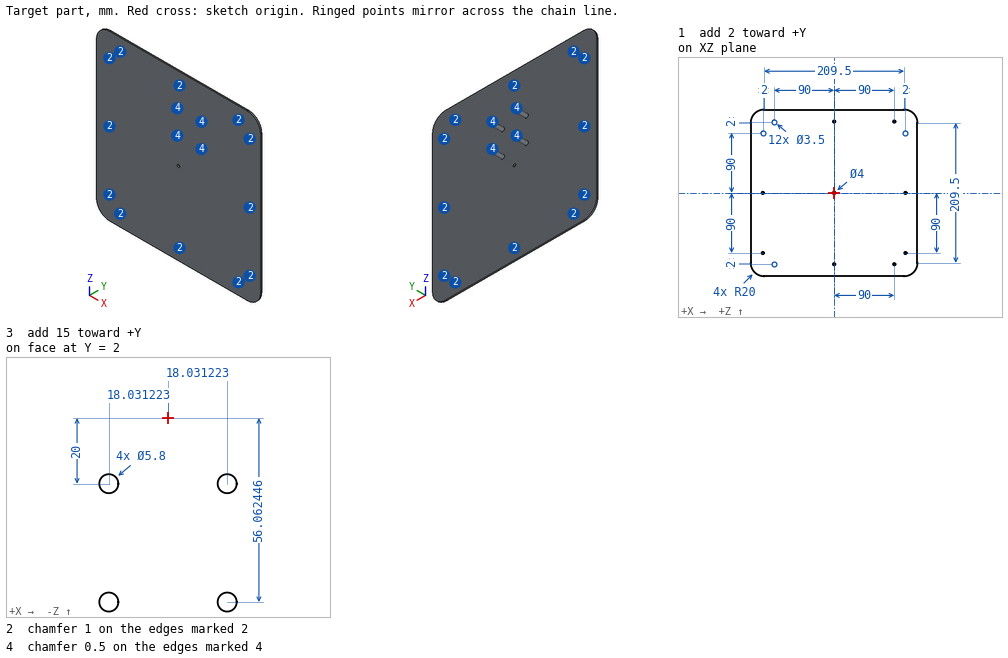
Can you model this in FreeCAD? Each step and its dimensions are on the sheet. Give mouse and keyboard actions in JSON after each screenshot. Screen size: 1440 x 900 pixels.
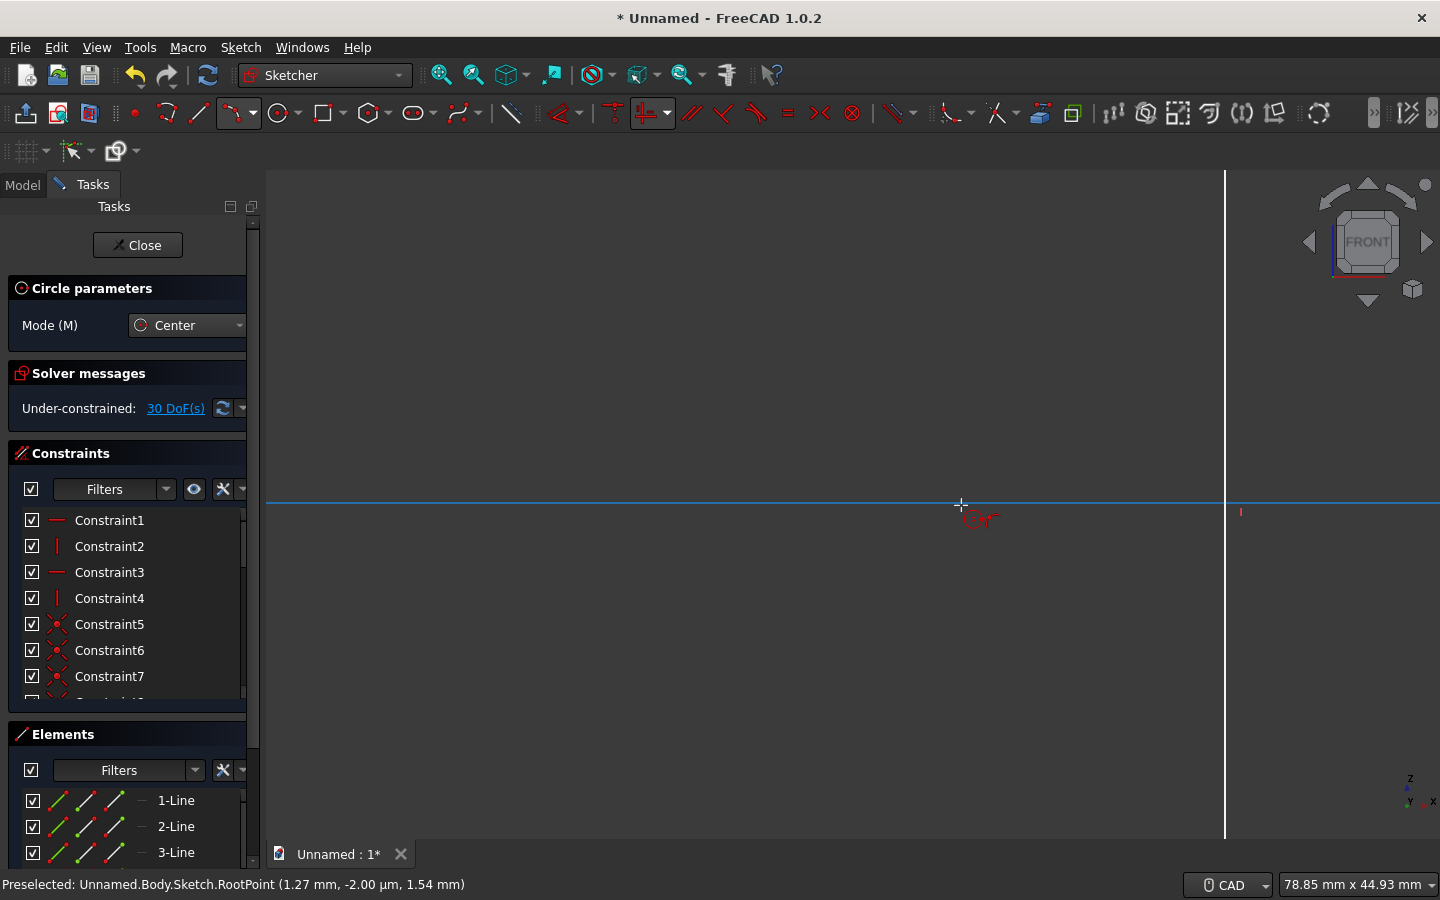
{"action": "scroll", "coordinate": [962, 505], "scroll_direction": "down", "scroll_amount": 11}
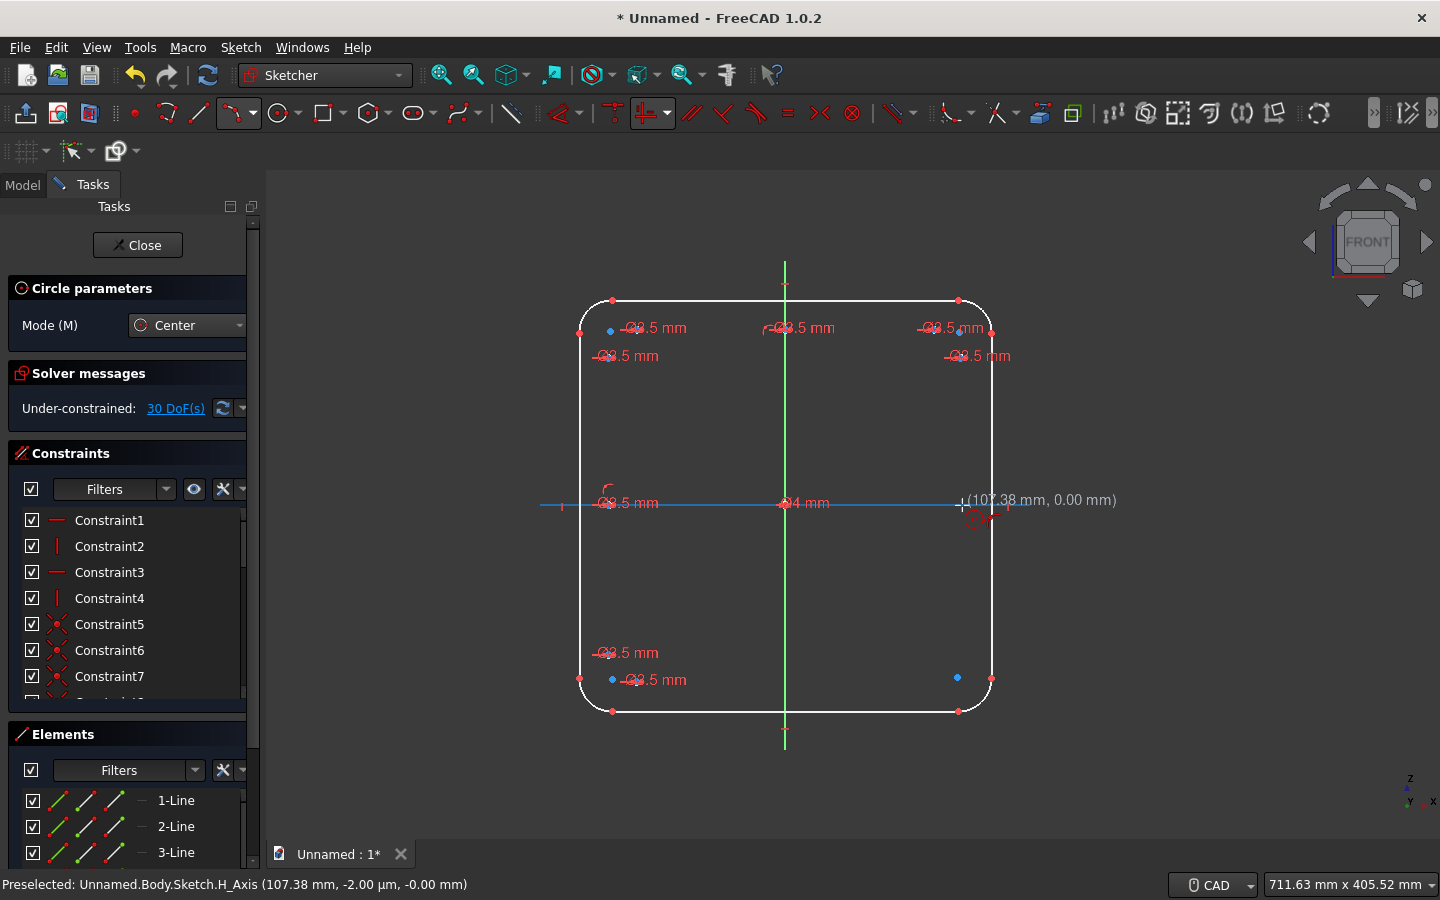
{"action": "left_click", "coordinate": [961, 505]}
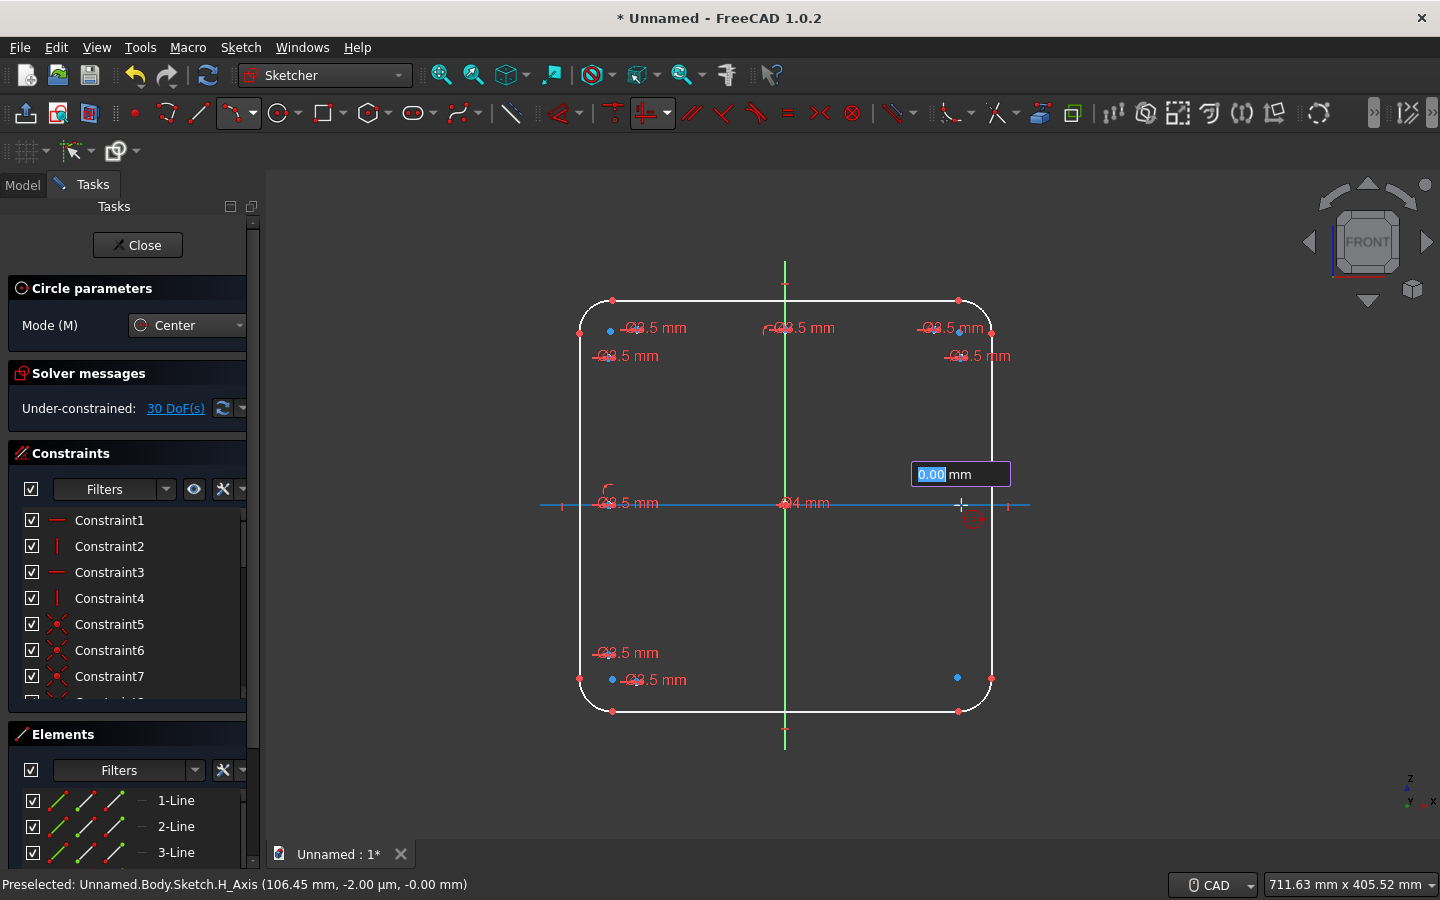
{"action": "scroll", "coordinate": [962, 502], "scroll_direction": "up", "scroll_amount": 9}
{"action": "mouse_move", "coordinate": [962, 502]}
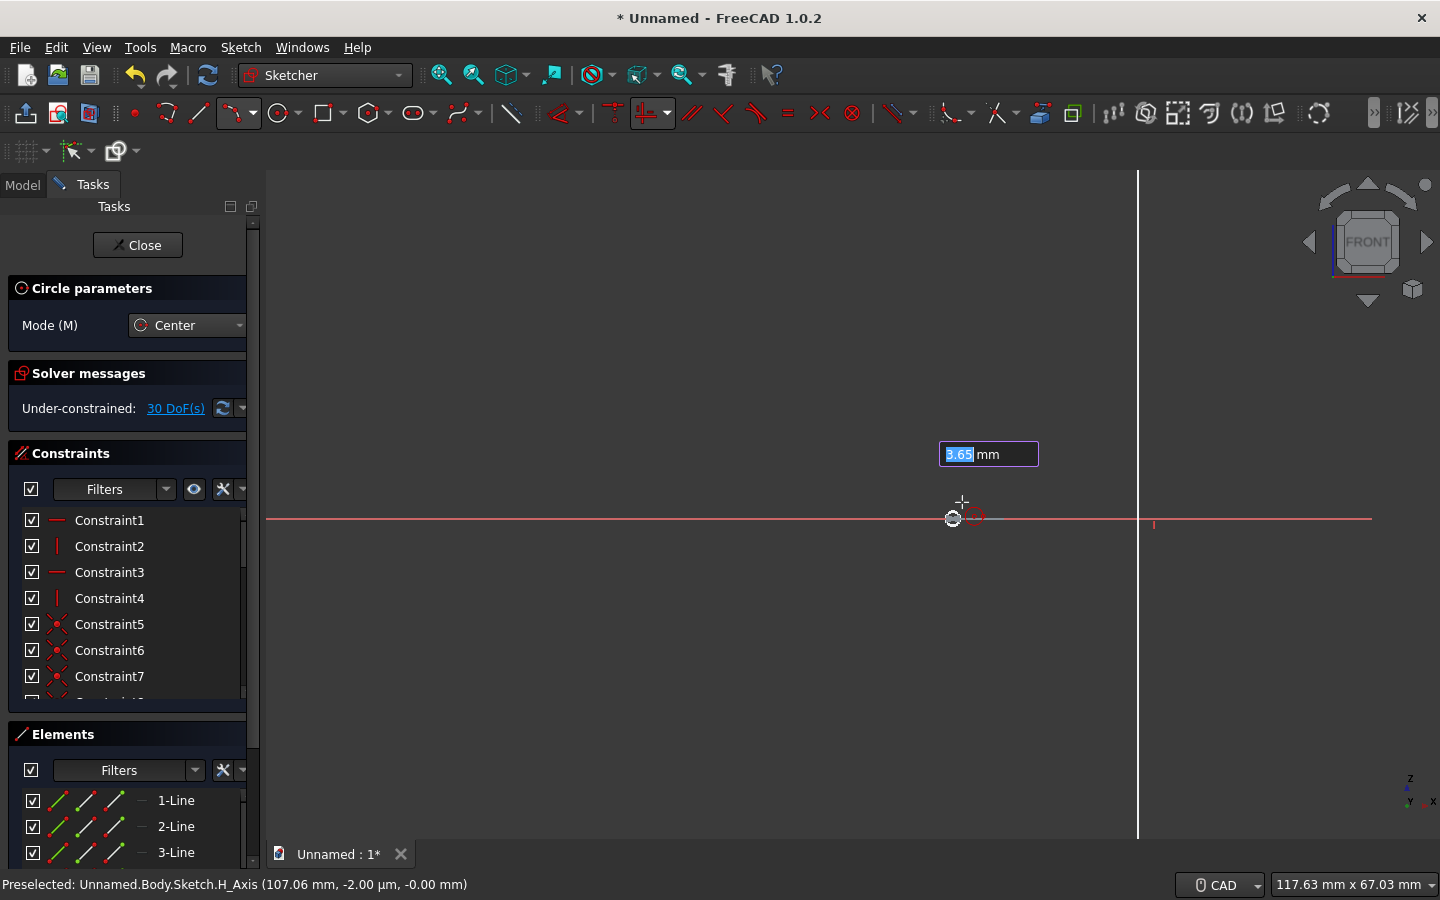
{"action": "type", "text": "3.5"}
{"action": "key", "text": "Return"}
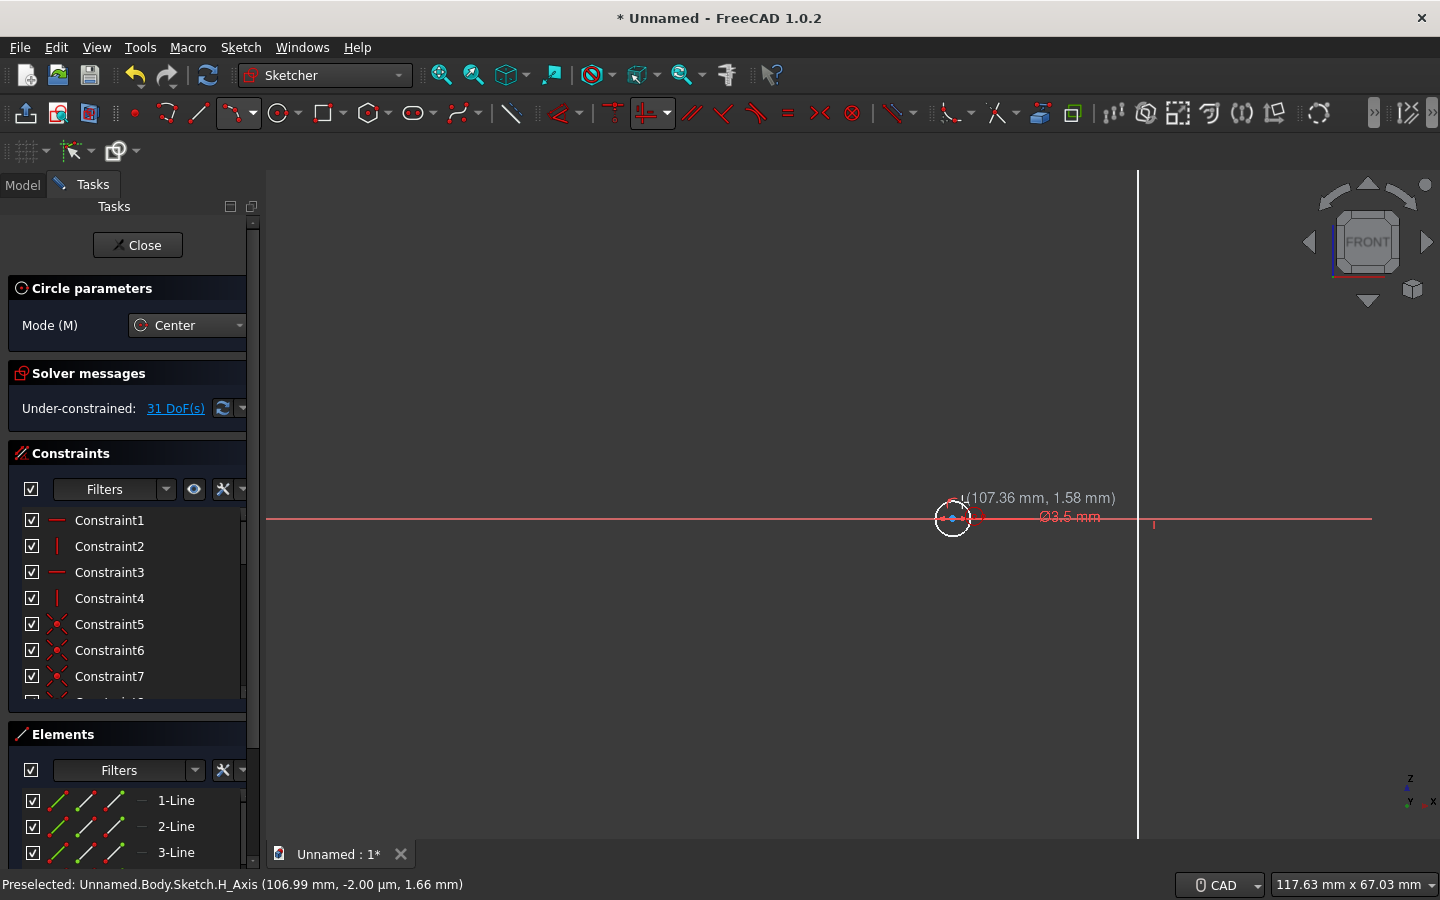
{"action": "scroll", "coordinate": [962, 502], "scroll_direction": "down", "scroll_amount": 9}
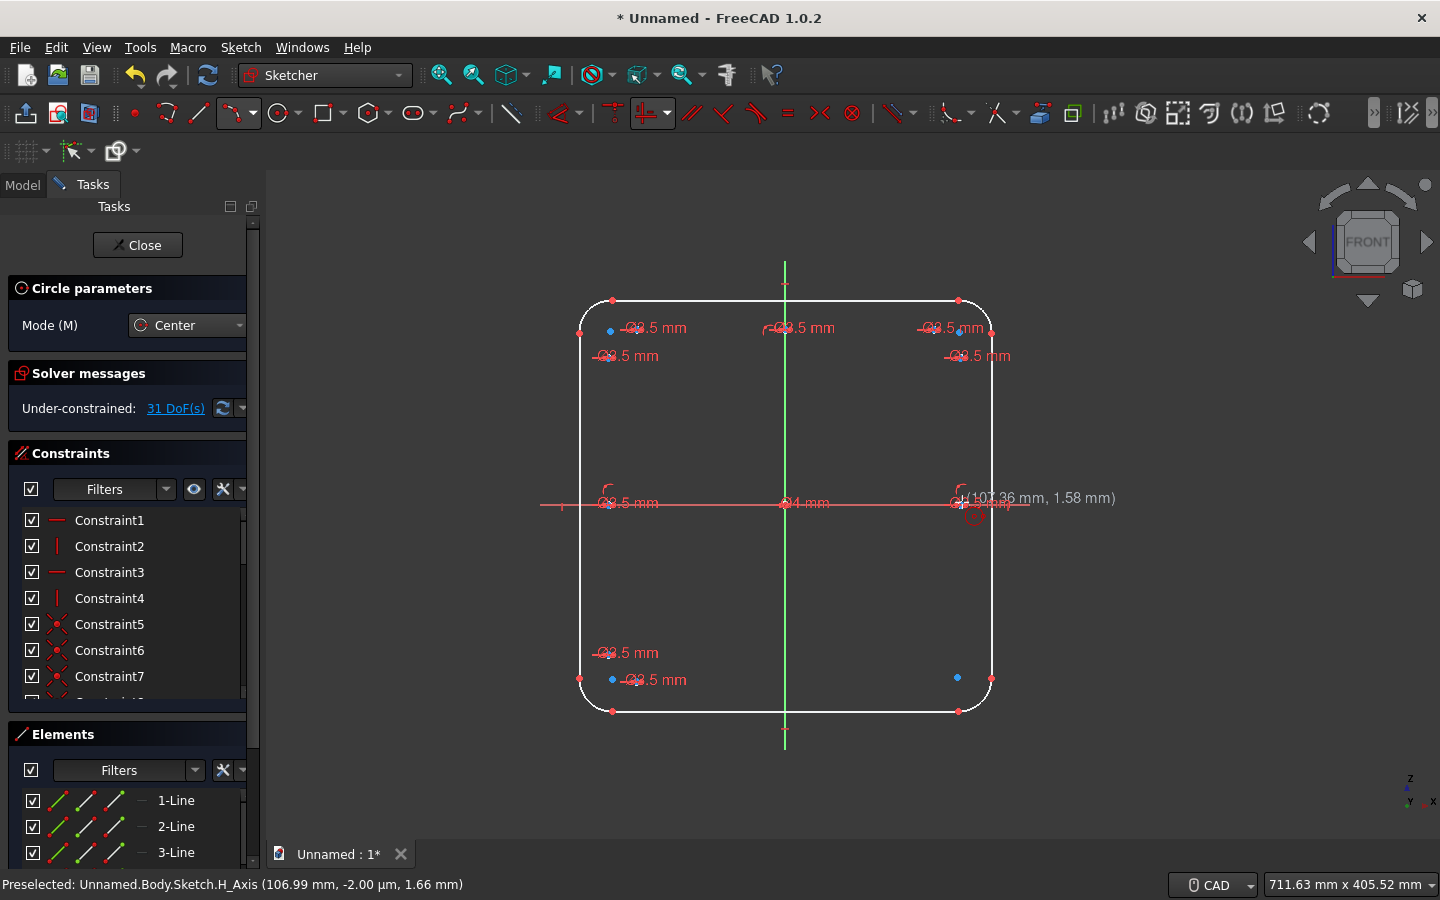
{"action": "scroll", "coordinate": [785, 681], "scroll_direction": "up", "scroll_amount": 11}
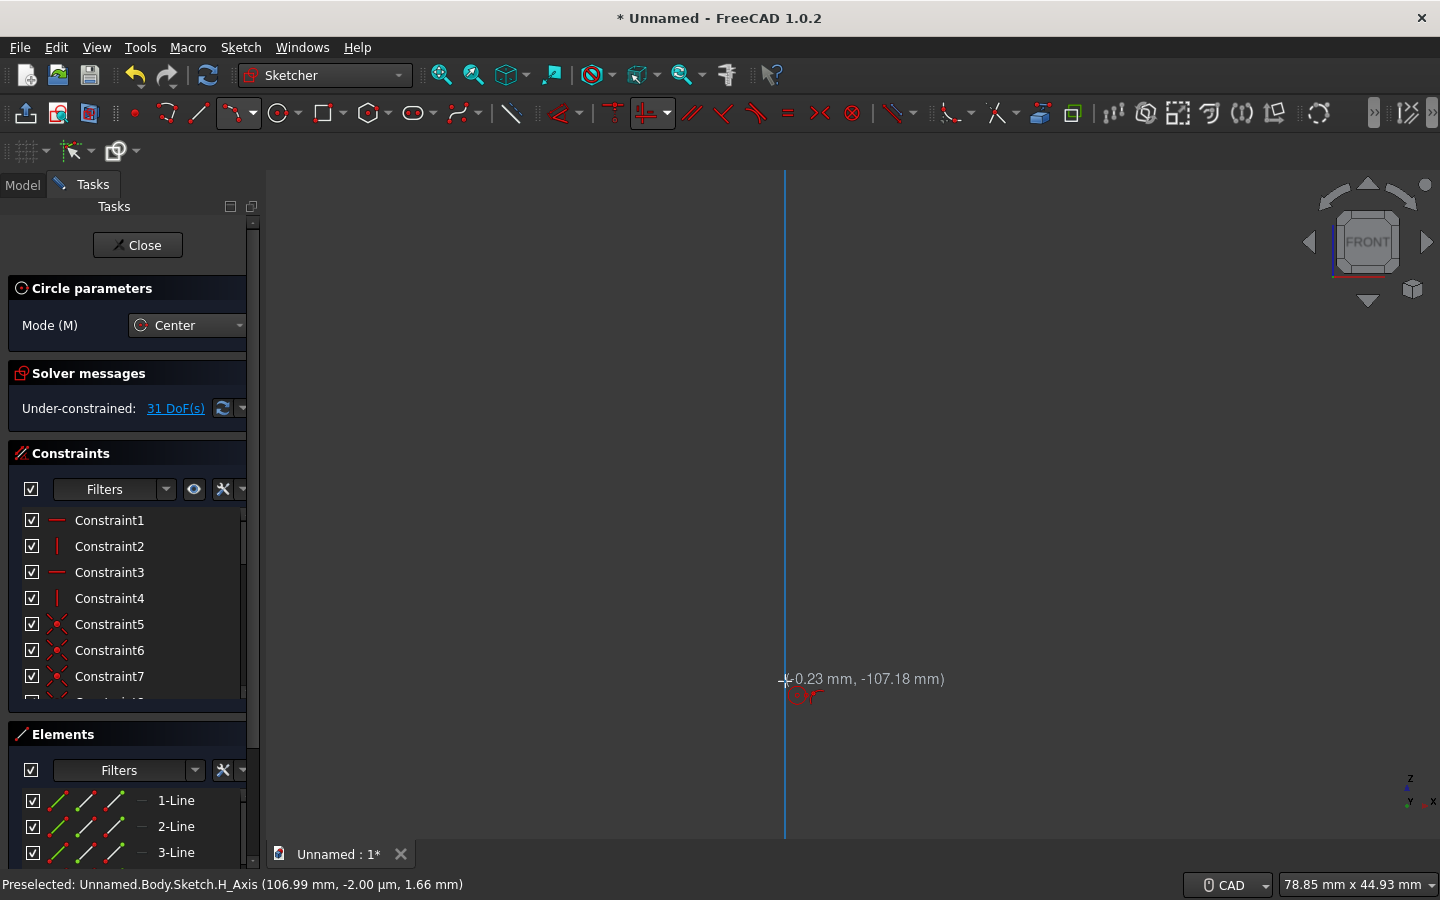
{"action": "scroll", "coordinate": [784, 681], "scroll_direction": "down", "scroll_amount": 11}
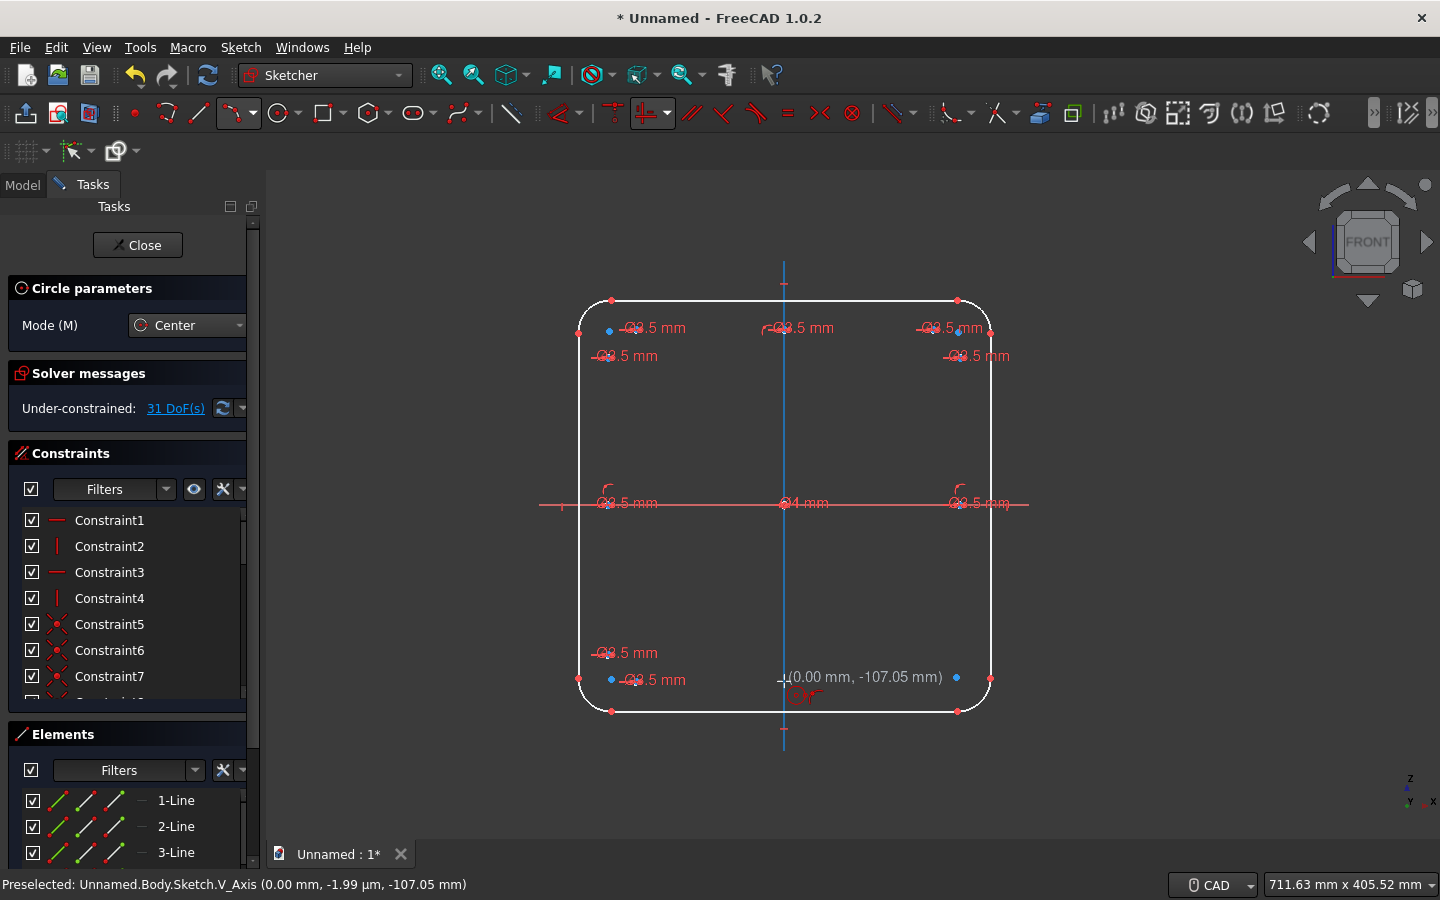
{"action": "left_click", "coordinate": [784, 681]}